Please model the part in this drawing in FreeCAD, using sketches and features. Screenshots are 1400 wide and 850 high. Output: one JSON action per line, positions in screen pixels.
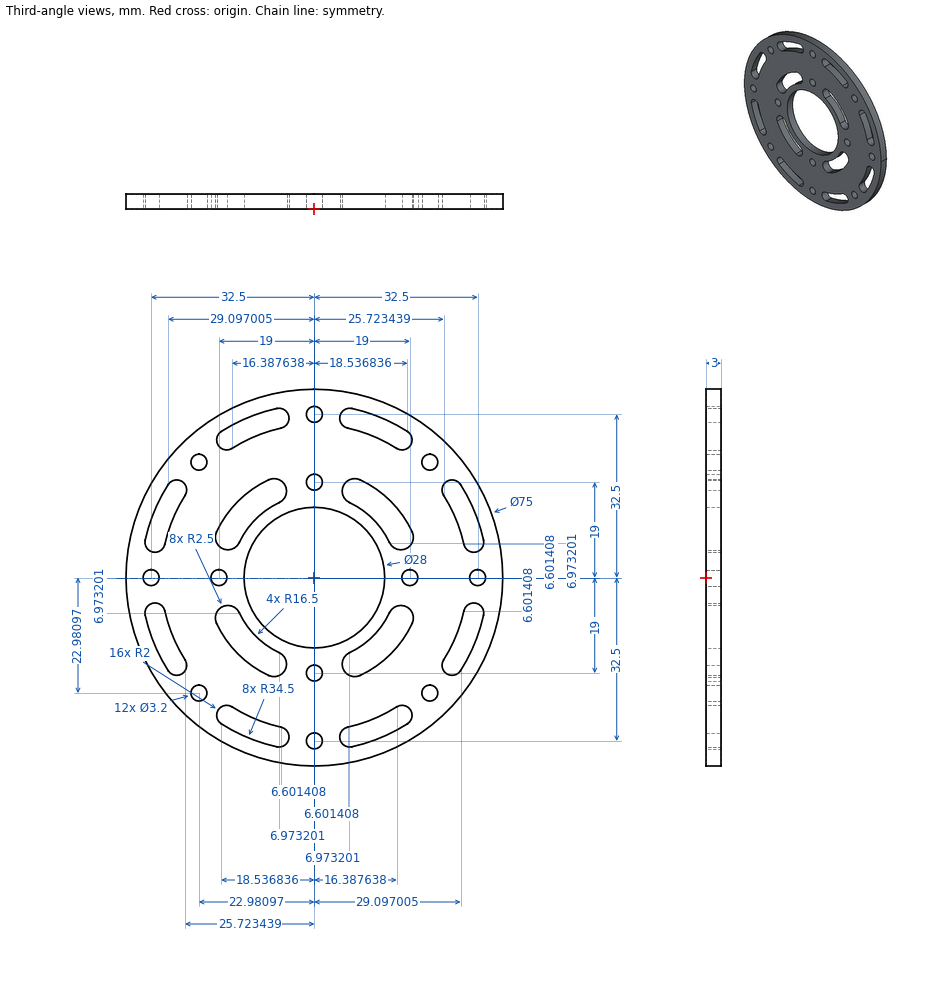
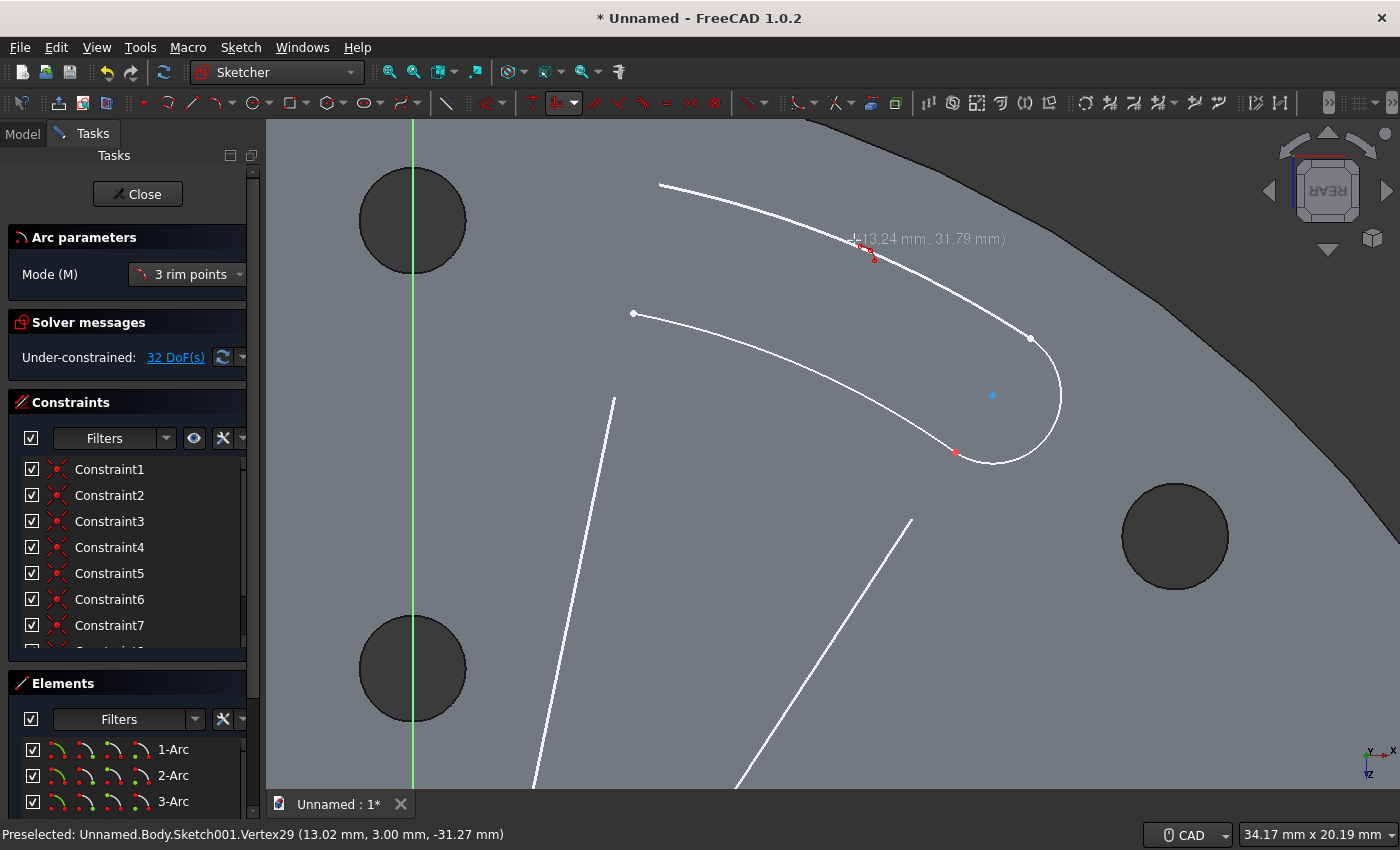
{"action": "left_click", "coordinate": [851, 241]}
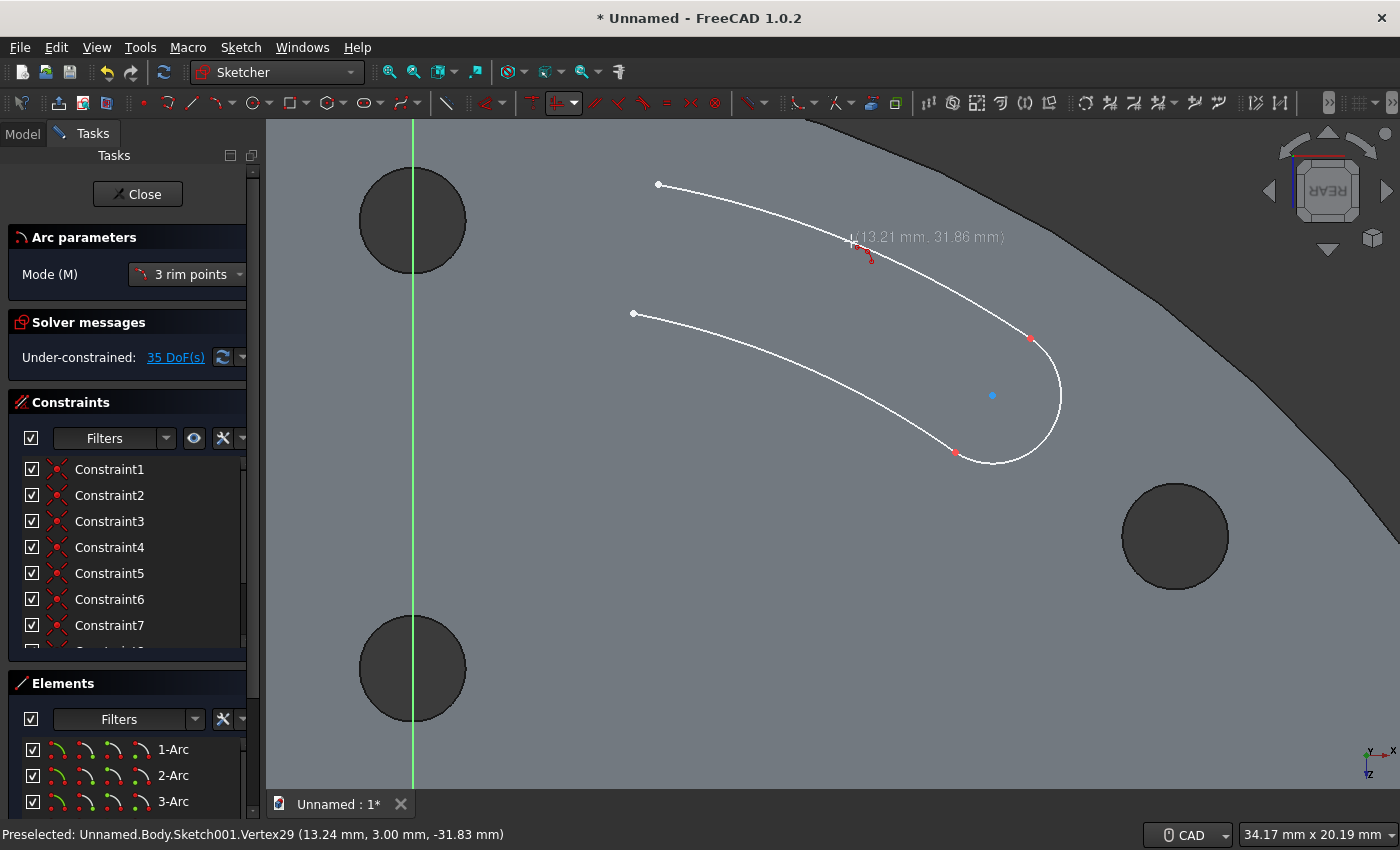
{"action": "scroll", "coordinate": [854, 240], "scroll_direction": "down", "scroll_amount": 8}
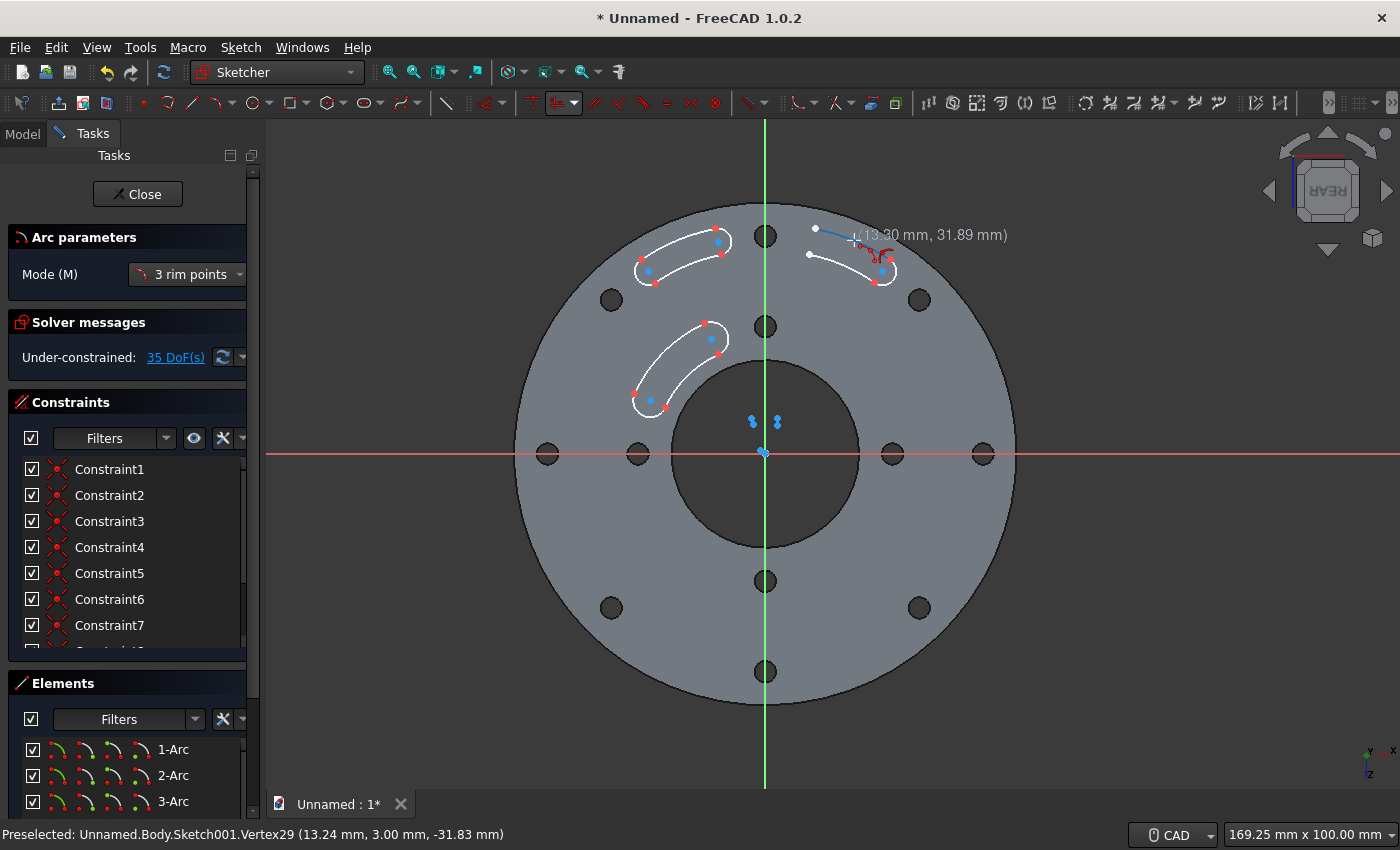
{"action": "left_click", "coordinate": [815, 229]}
{"action": "left_click", "coordinate": [810, 255]}
{"action": "left_click", "coordinate": [799, 239]}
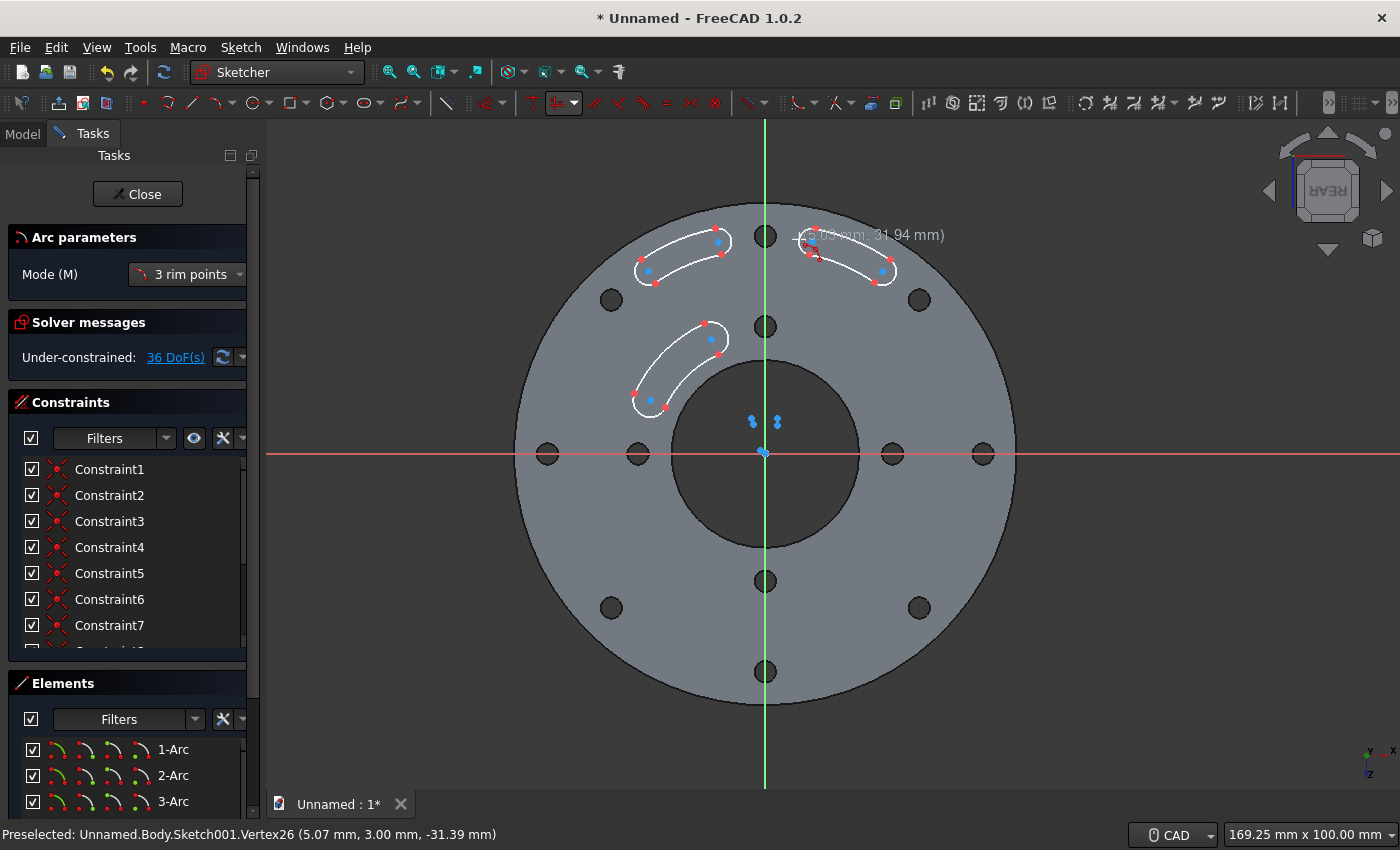
{"action": "left_click", "coordinate": [965, 410]}
{"action": "left_click", "coordinate": [991, 404]}
{"action": "left_click", "coordinate": [981, 420]}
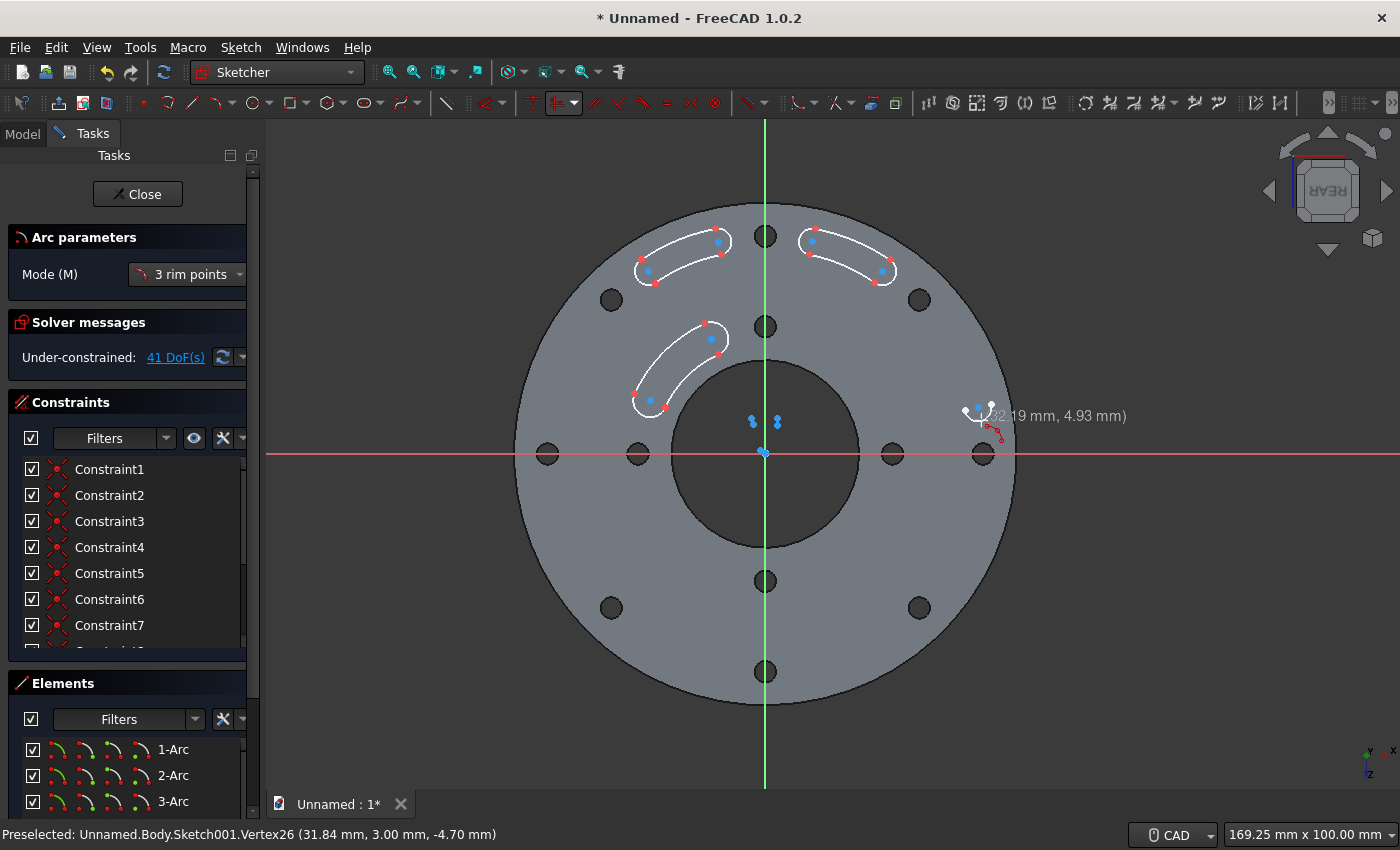
{"action": "left_click", "coordinate": [991, 405]}
{"action": "left_click", "coordinate": [960, 330]}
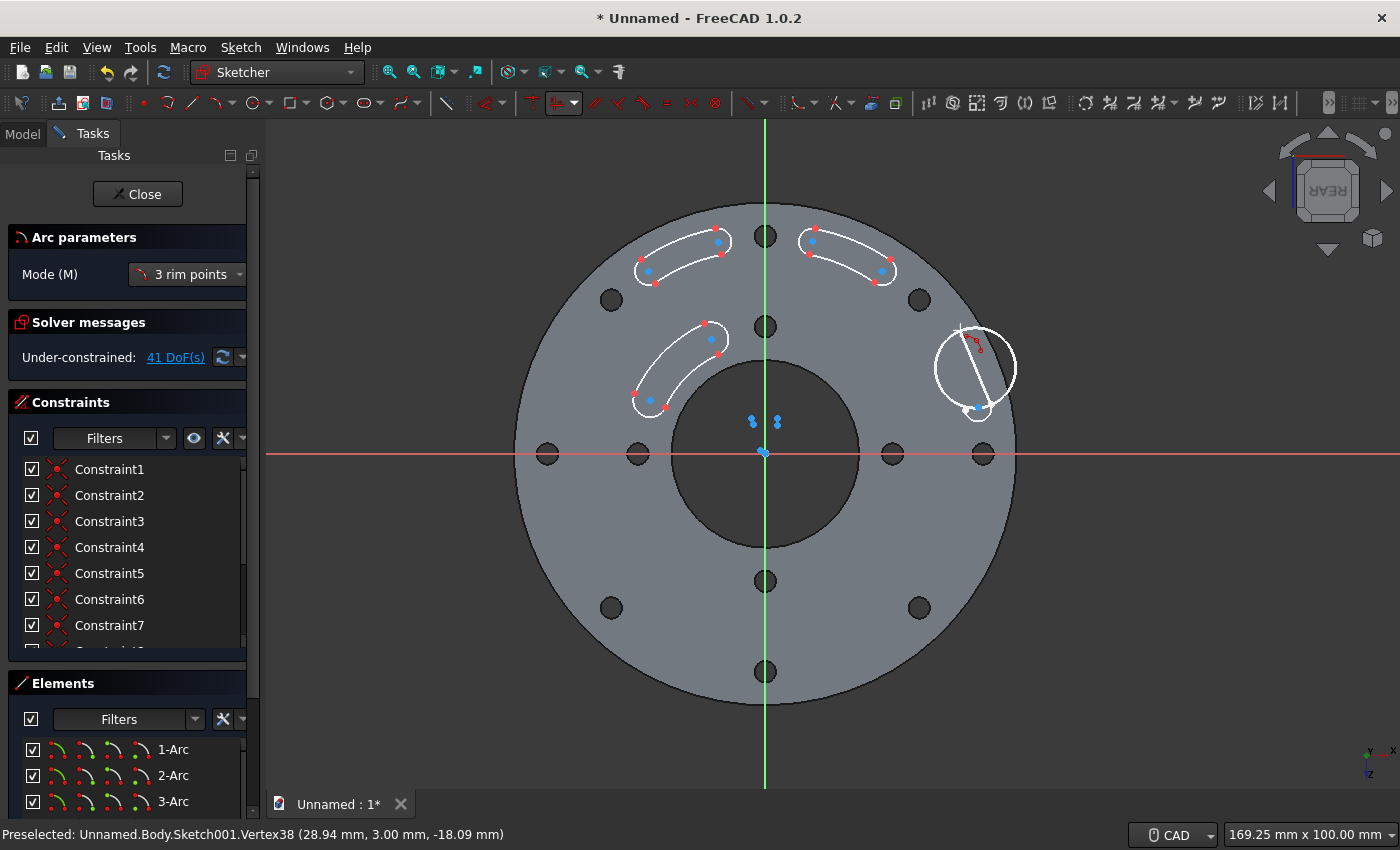
{"action": "scroll", "coordinate": [979, 366], "scroll_direction": "up", "scroll_amount": 8}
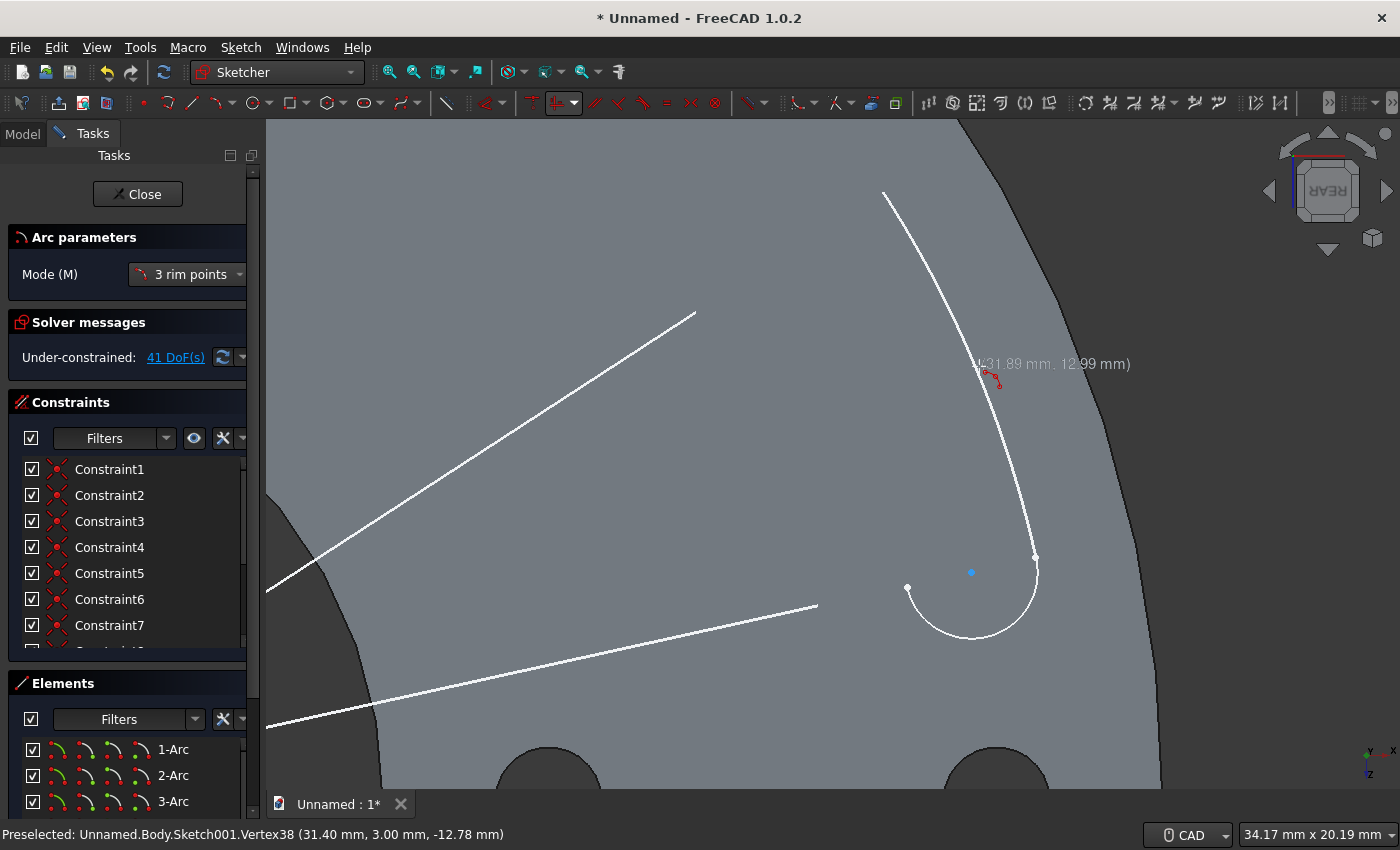
{"action": "left_click", "coordinate": [976, 362]}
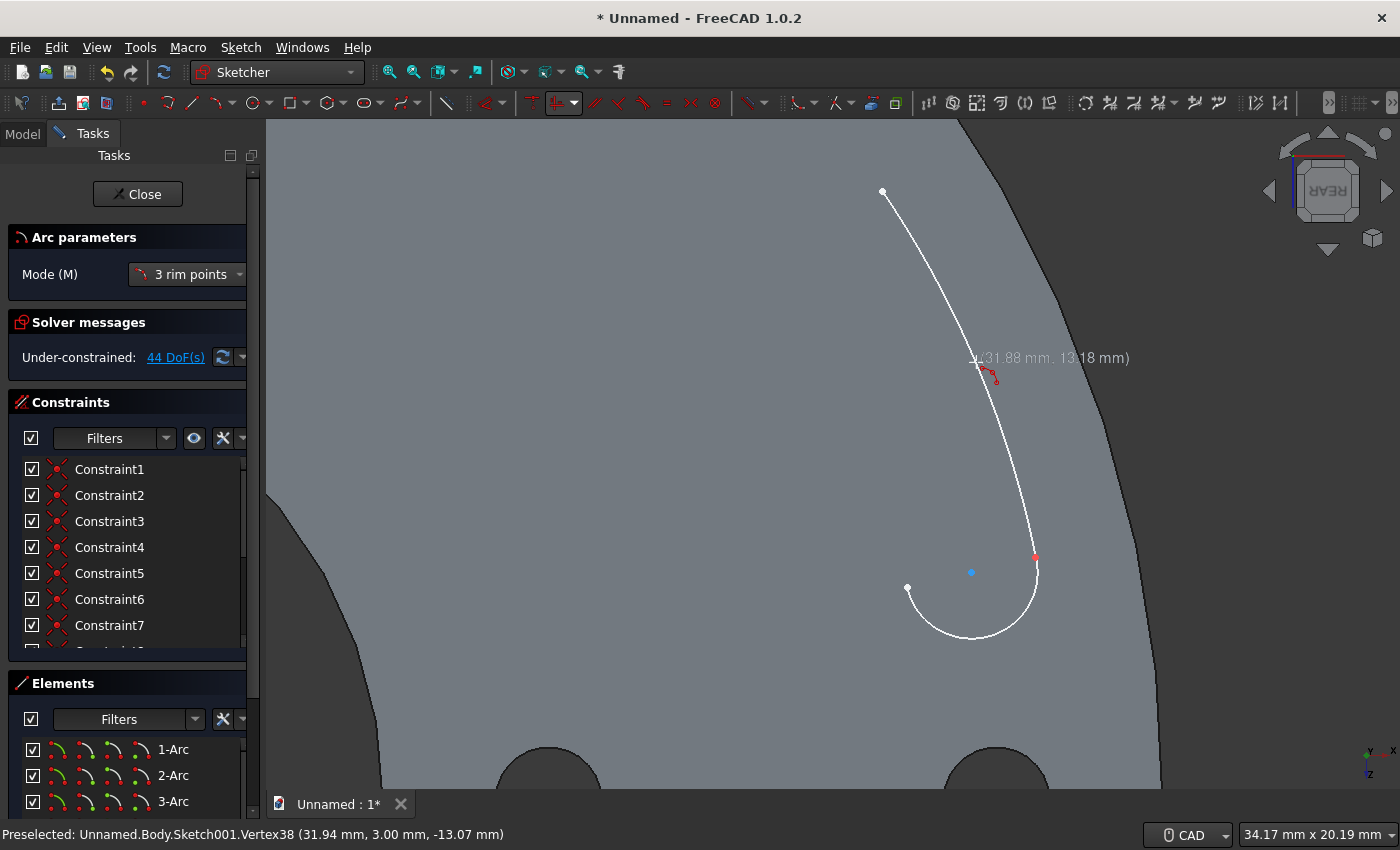
{"action": "scroll", "coordinate": [979, 366], "scroll_direction": "down", "scroll_amount": 8}